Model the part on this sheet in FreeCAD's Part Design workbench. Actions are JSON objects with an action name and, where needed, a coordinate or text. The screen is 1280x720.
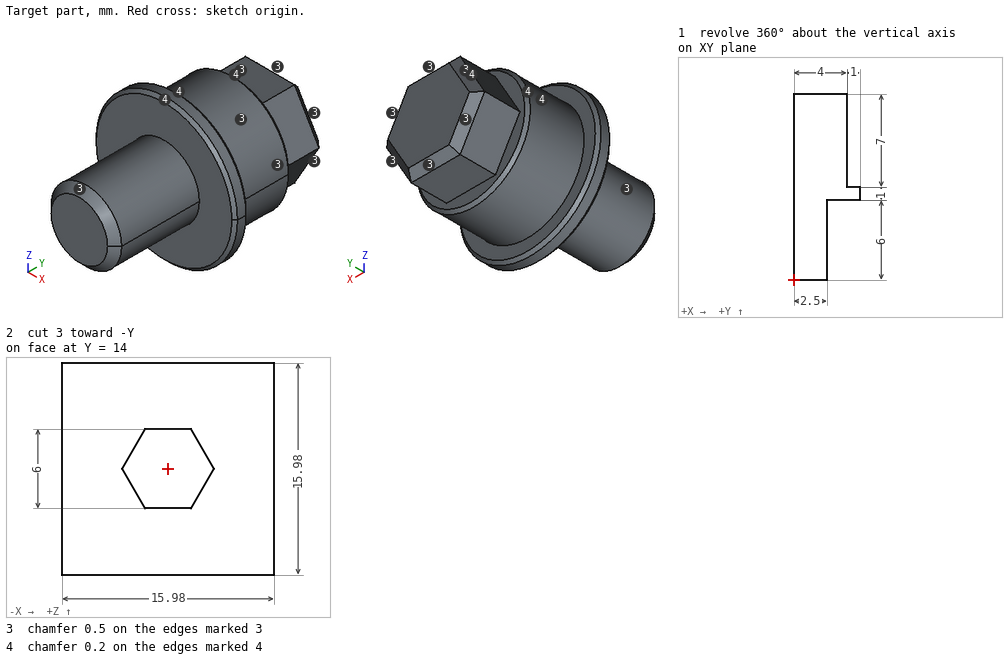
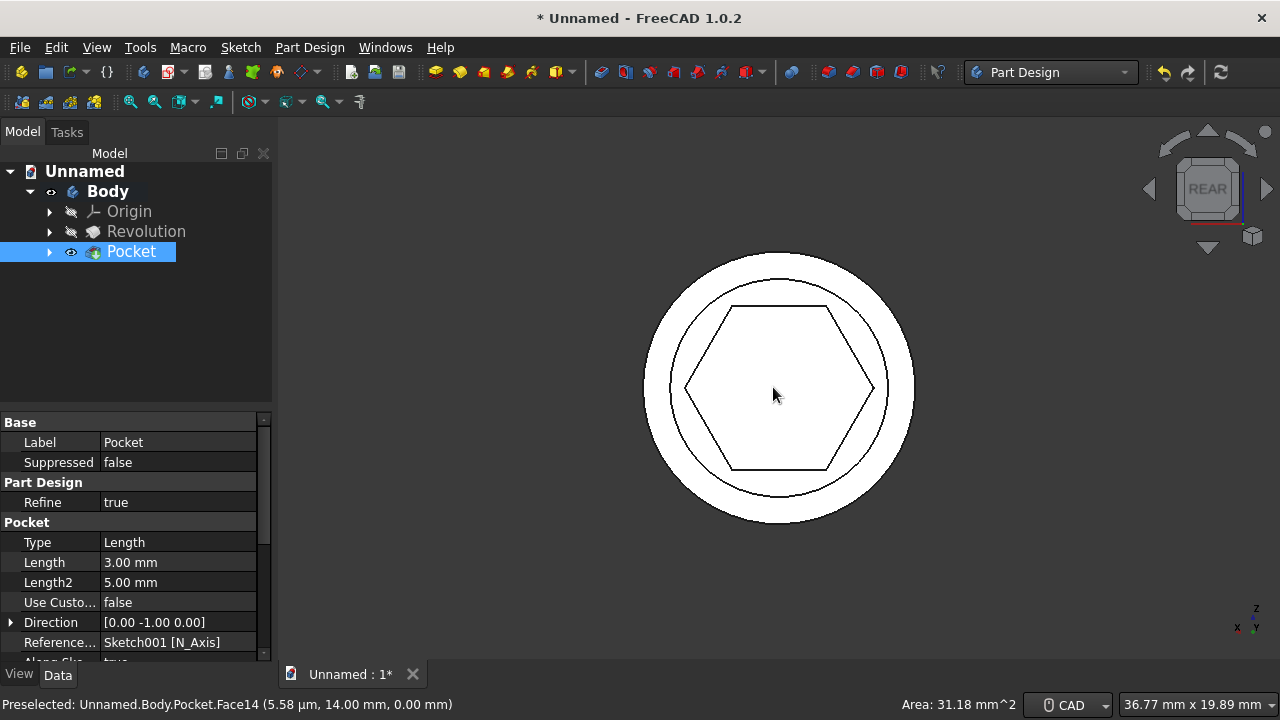
{"action": "key", "text": "0"}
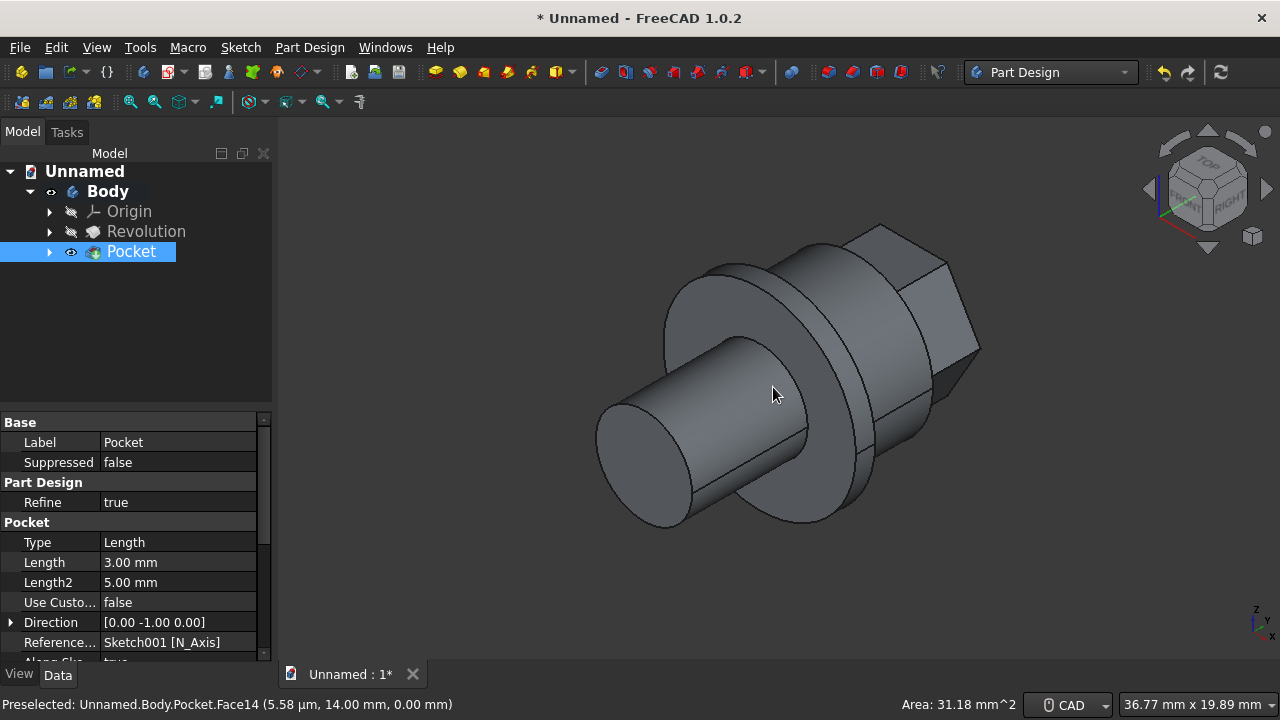
{"action": "left_click", "coordinate": [605, 410], "text": "ctrl"}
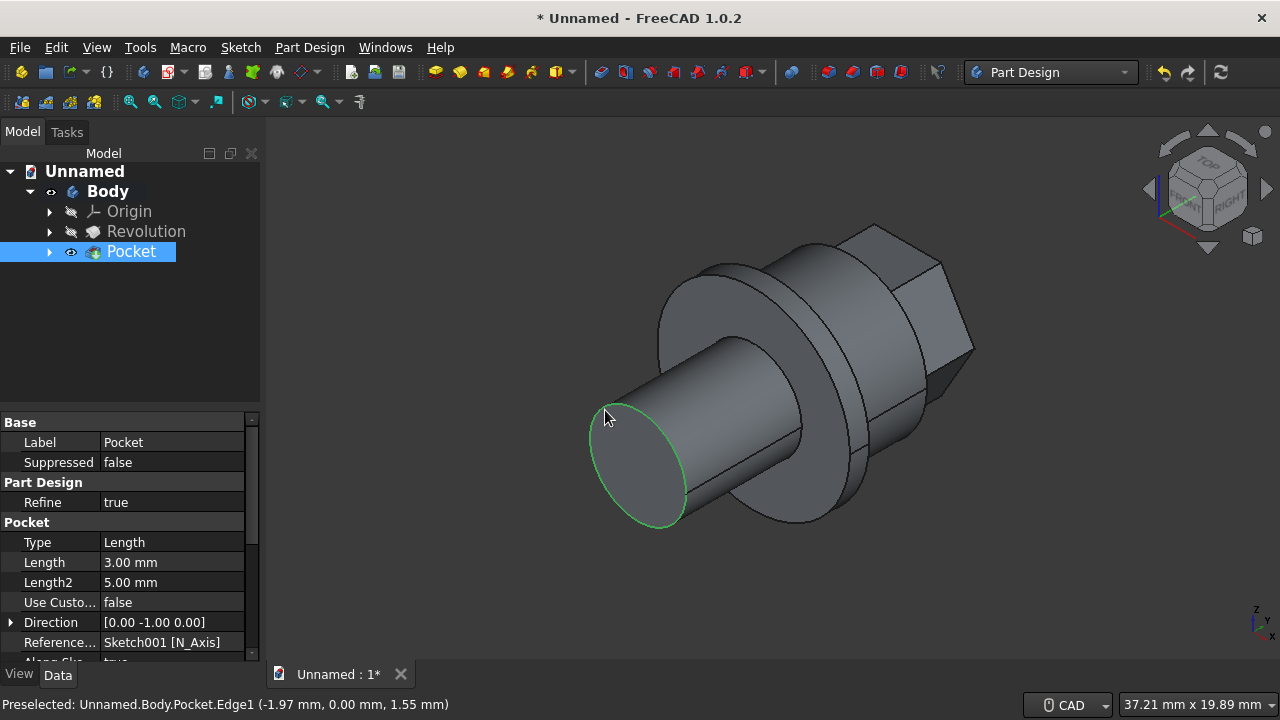
{"action": "left_click", "coordinate": [854, 72]}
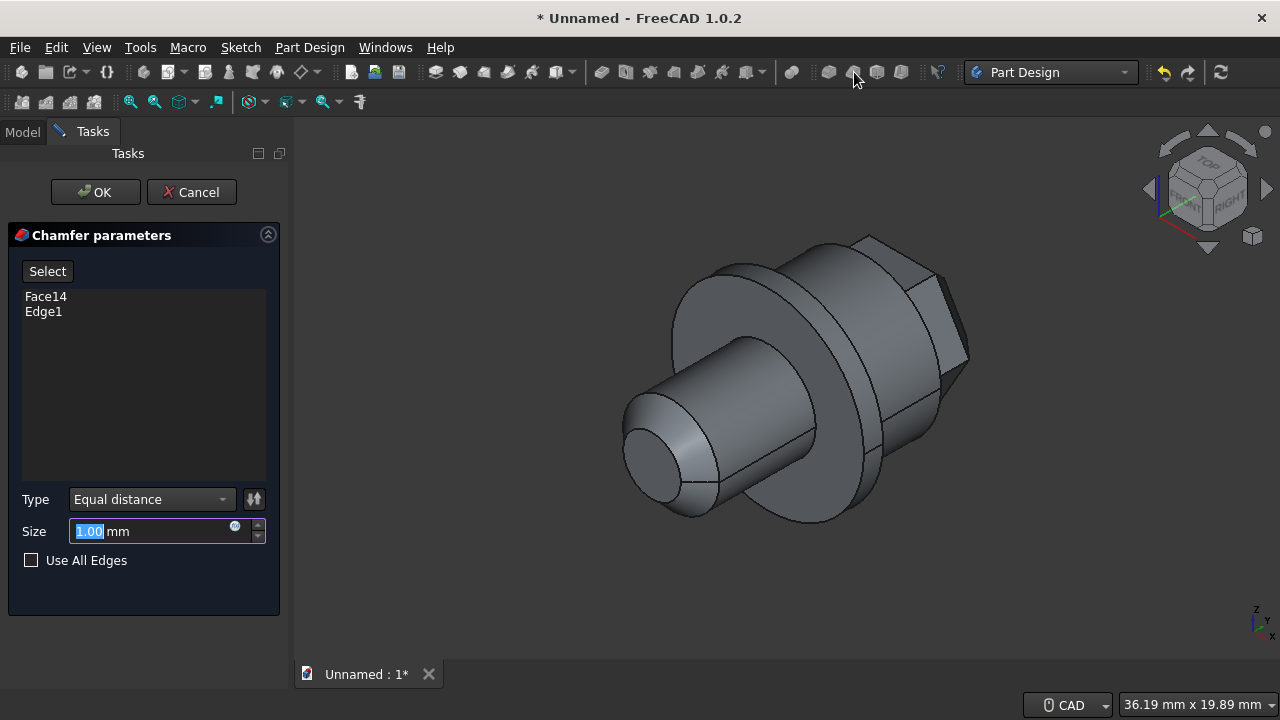
{"action": "type", "text": "0.5"}
{"action": "key", "text": "Tab"}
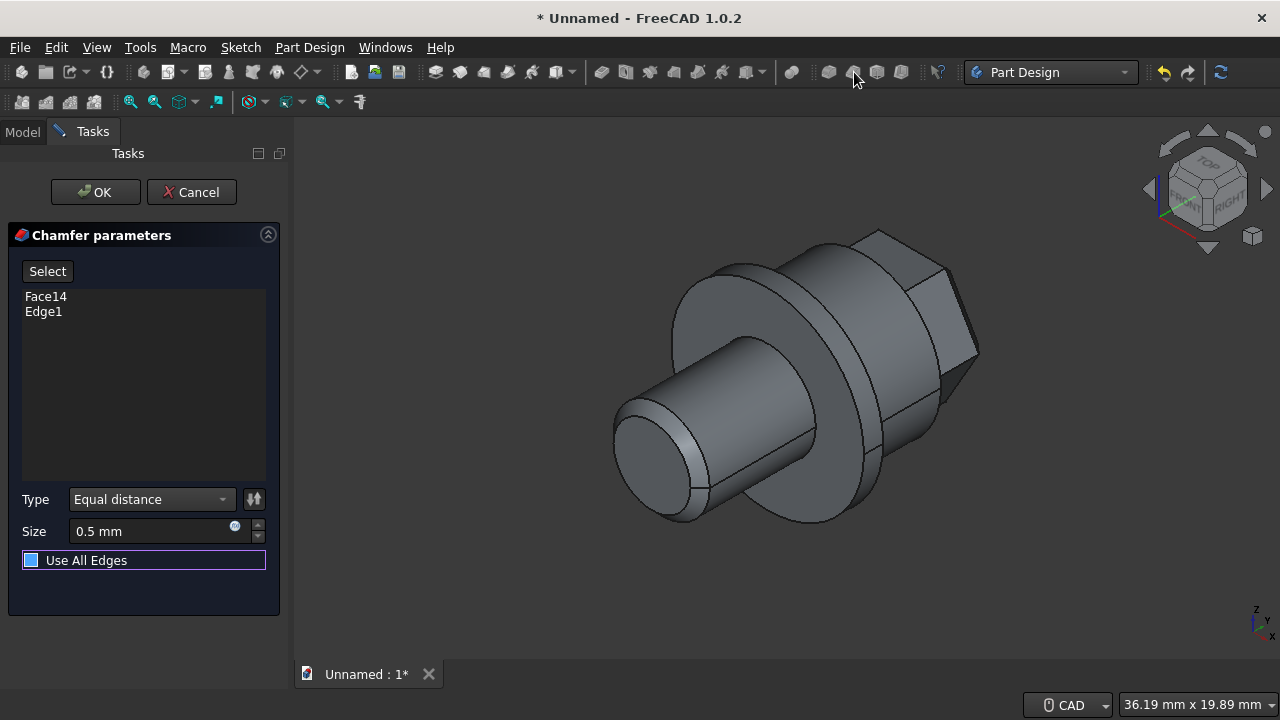
{"action": "left_click", "coordinate": [96, 192]}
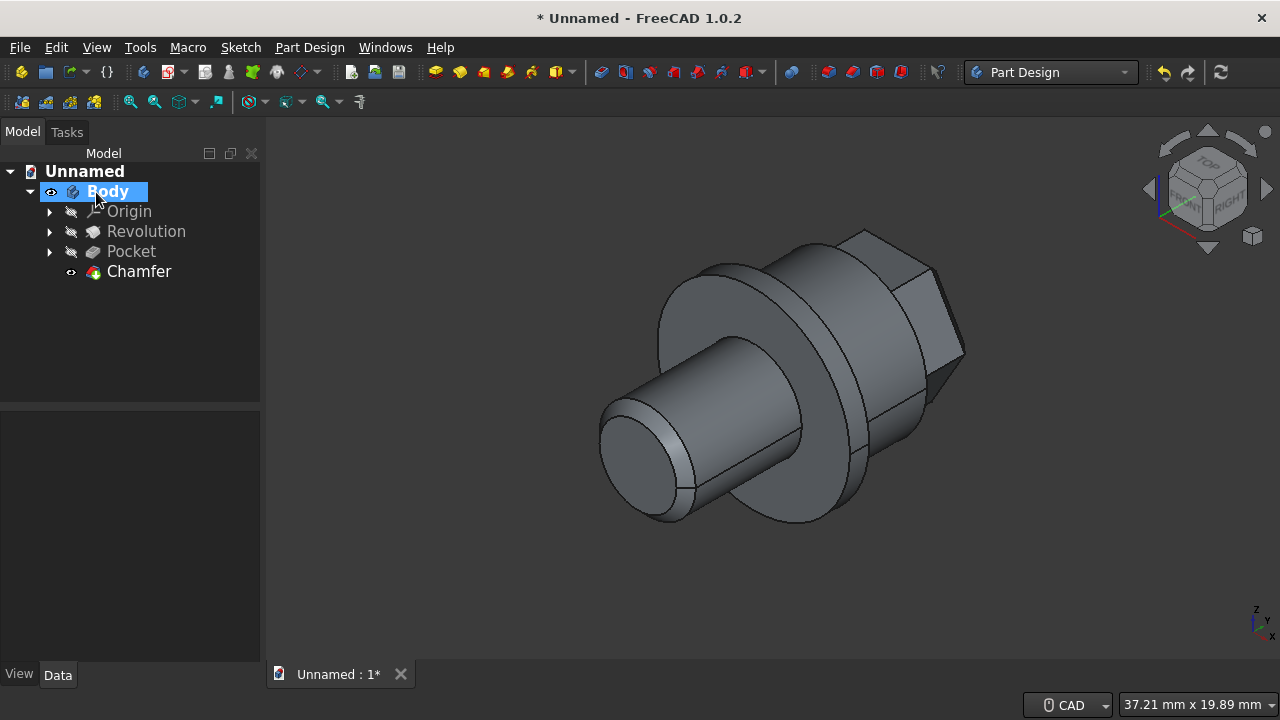
{"action": "left_click", "coordinate": [724, 275]}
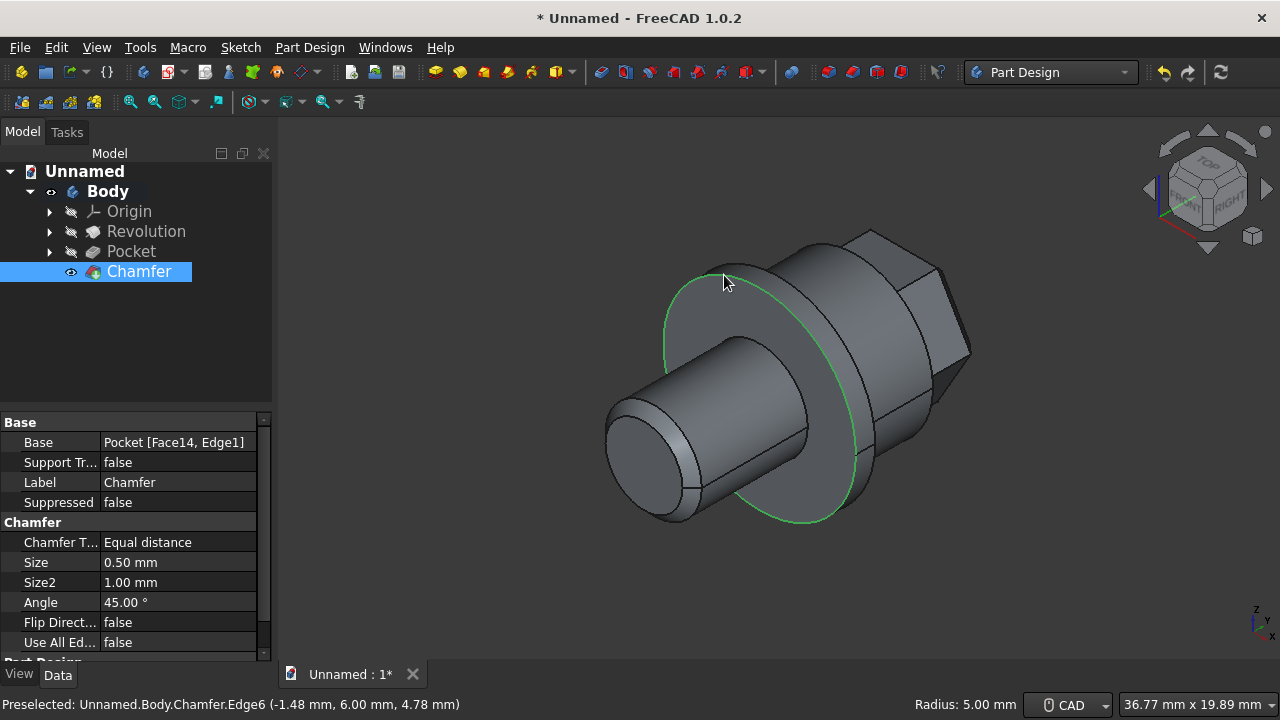
{"action": "key", "text": "2"}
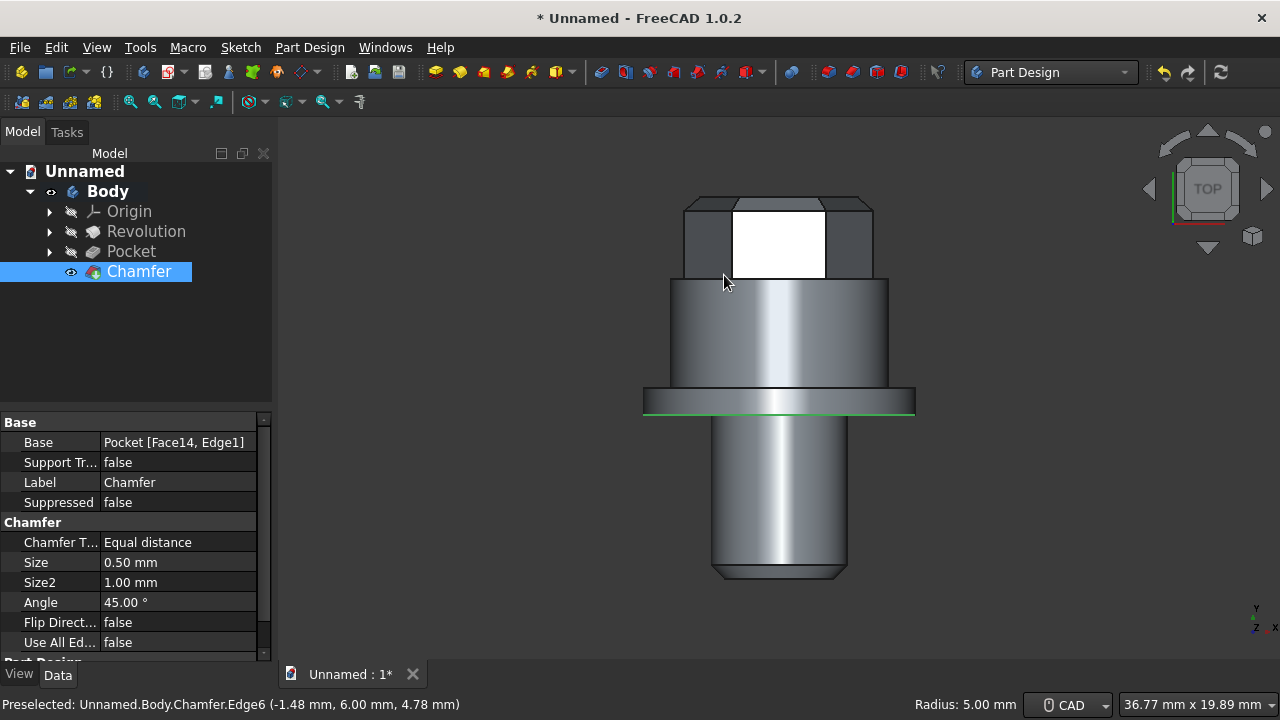
{"action": "left_click", "coordinate": [691, 278], "text": "ctrl"}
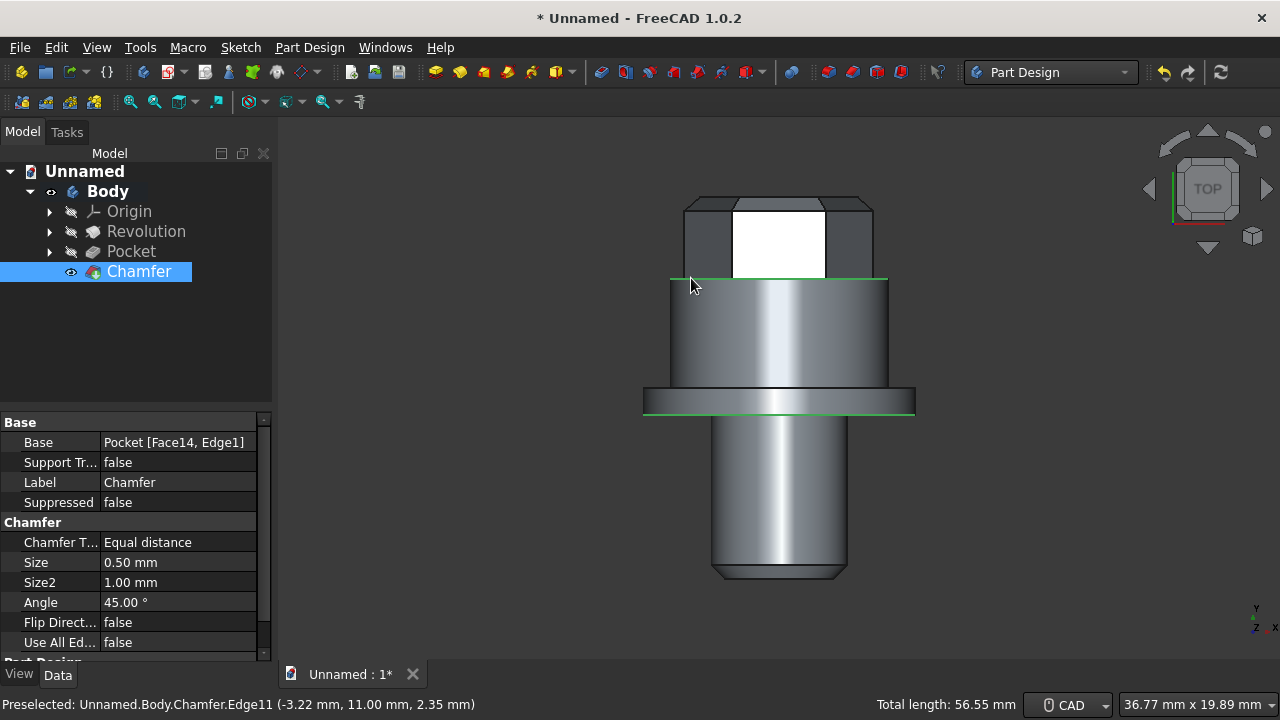
{"action": "left_click", "coordinate": [669, 387], "text": "ctrl"}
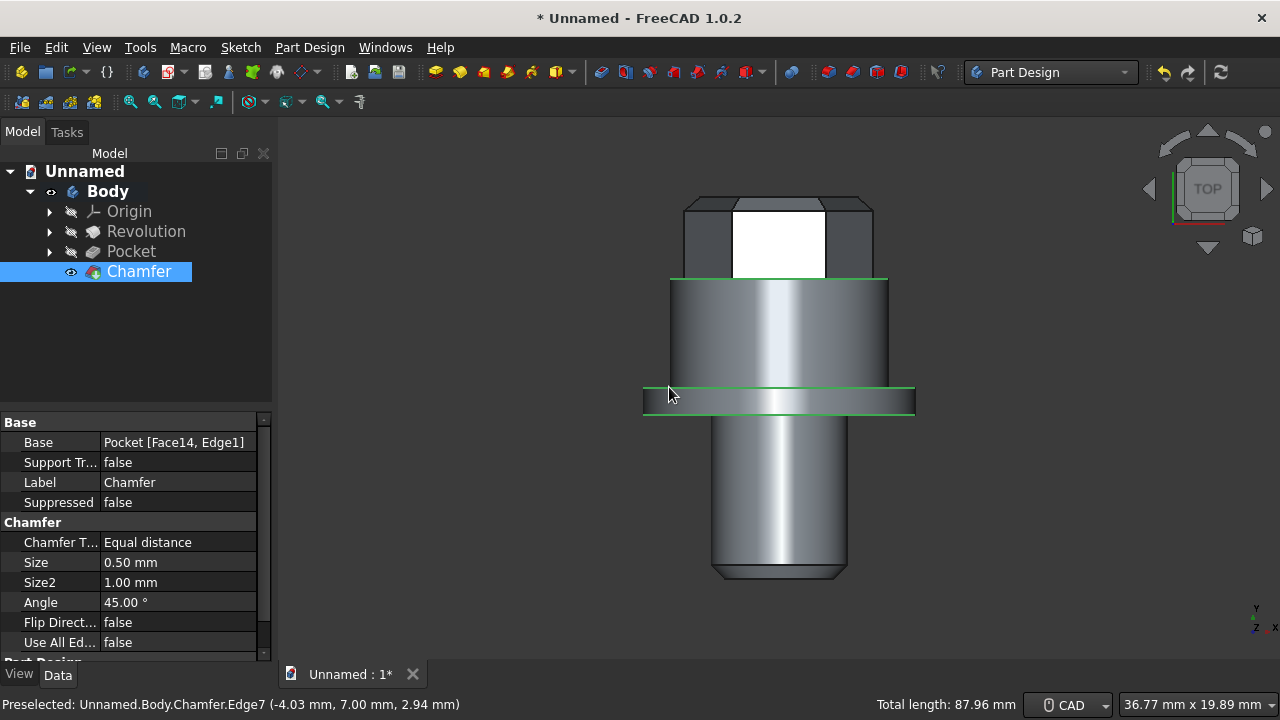
{"action": "left_click", "coordinate": [854, 72]}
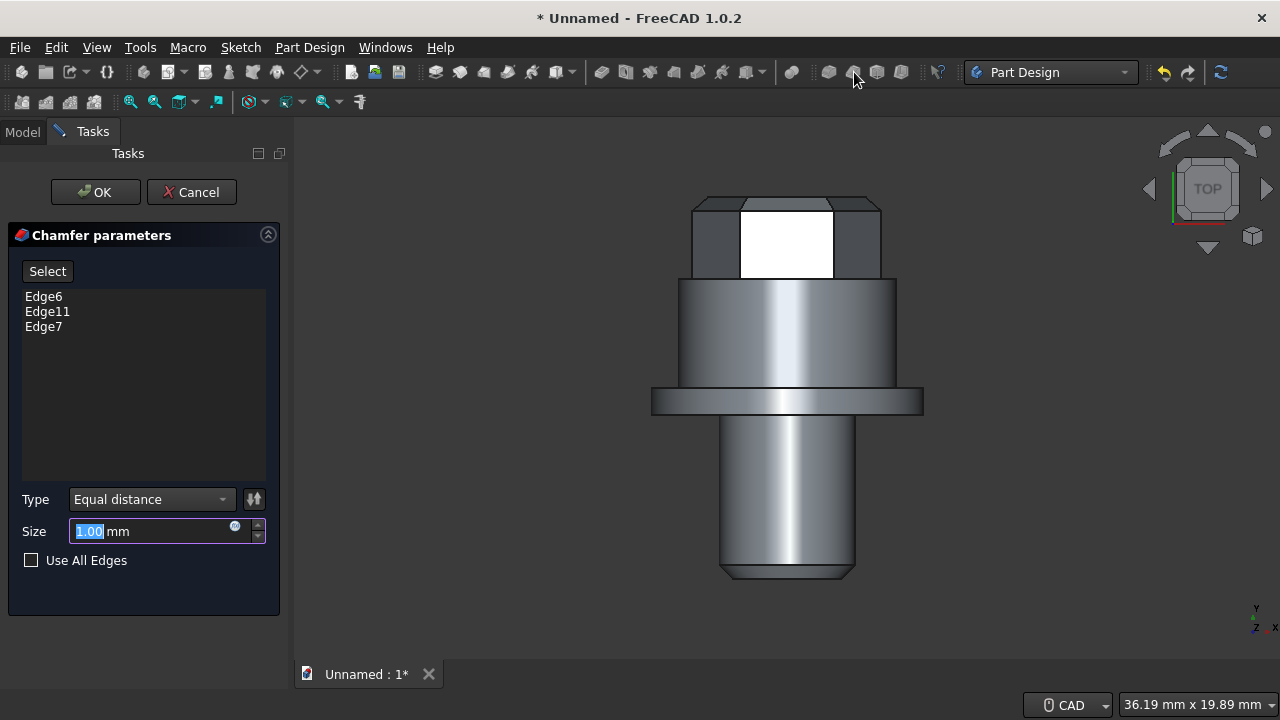
{"action": "type", "text": "0.2"}
{"action": "key", "text": "Tab"}